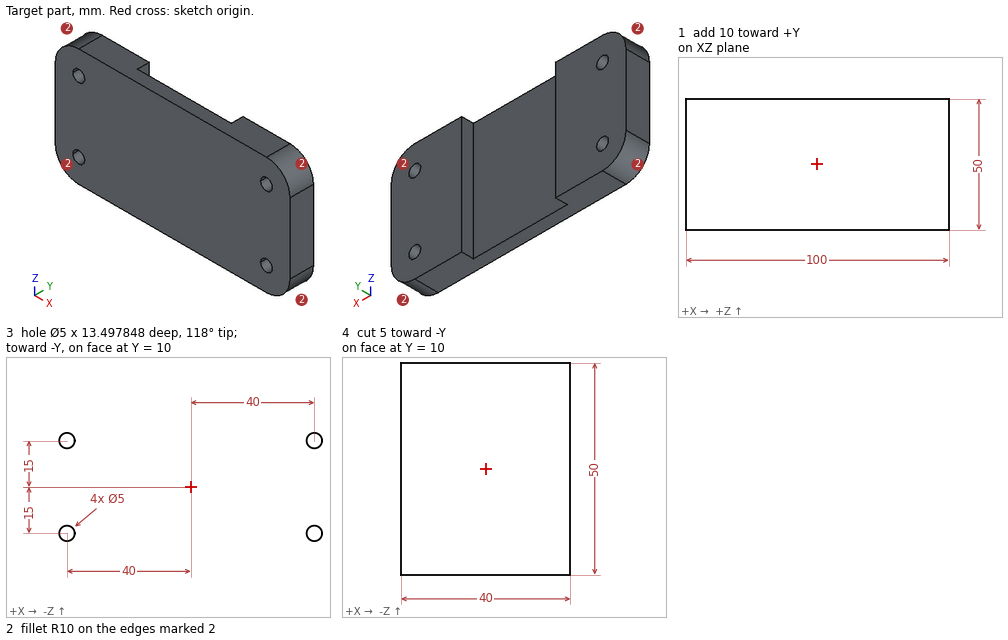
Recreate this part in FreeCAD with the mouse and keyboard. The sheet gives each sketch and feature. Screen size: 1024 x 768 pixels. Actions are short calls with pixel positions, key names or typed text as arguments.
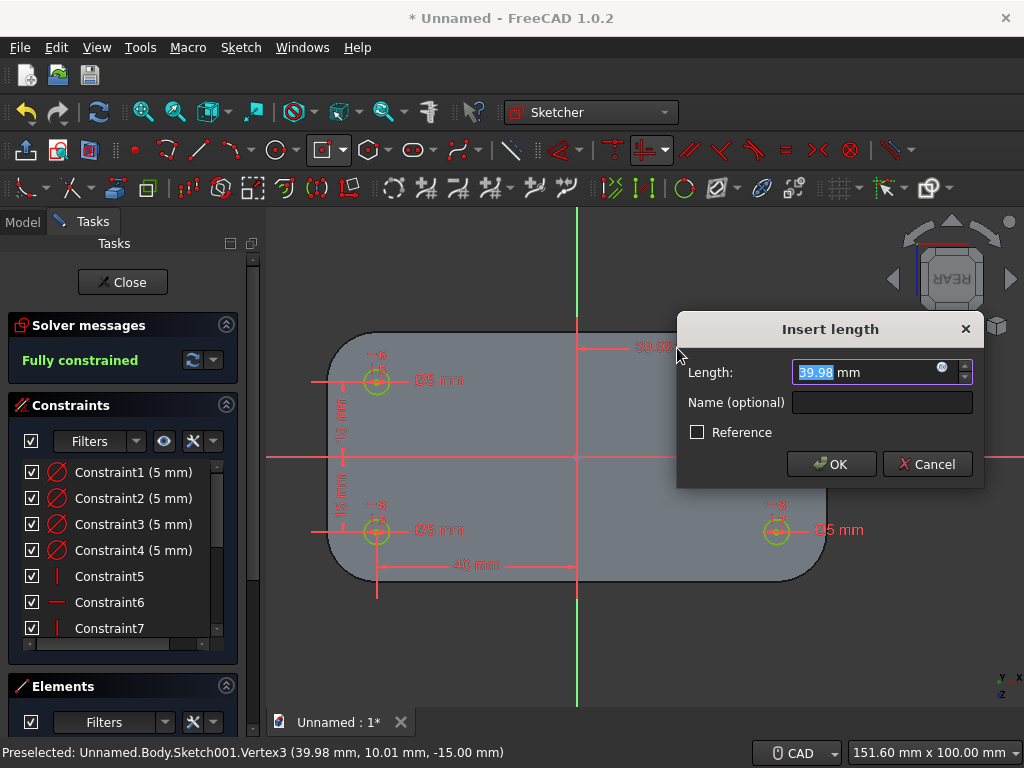
text(40)
key(Return)
key(Escape)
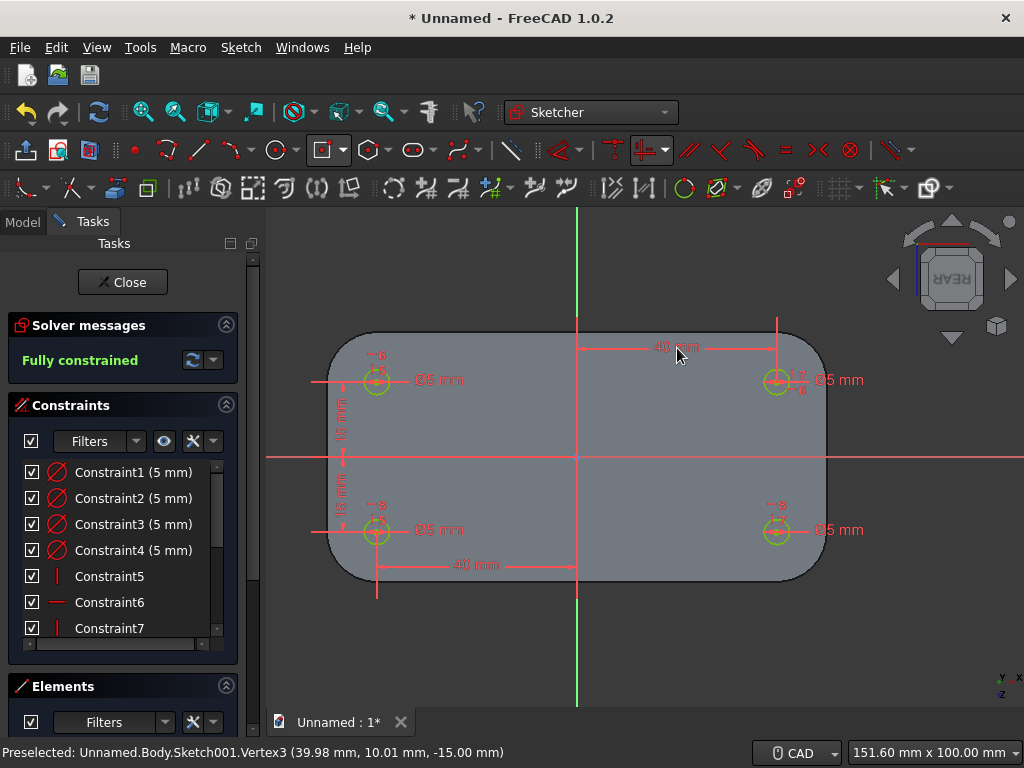
click(123, 282)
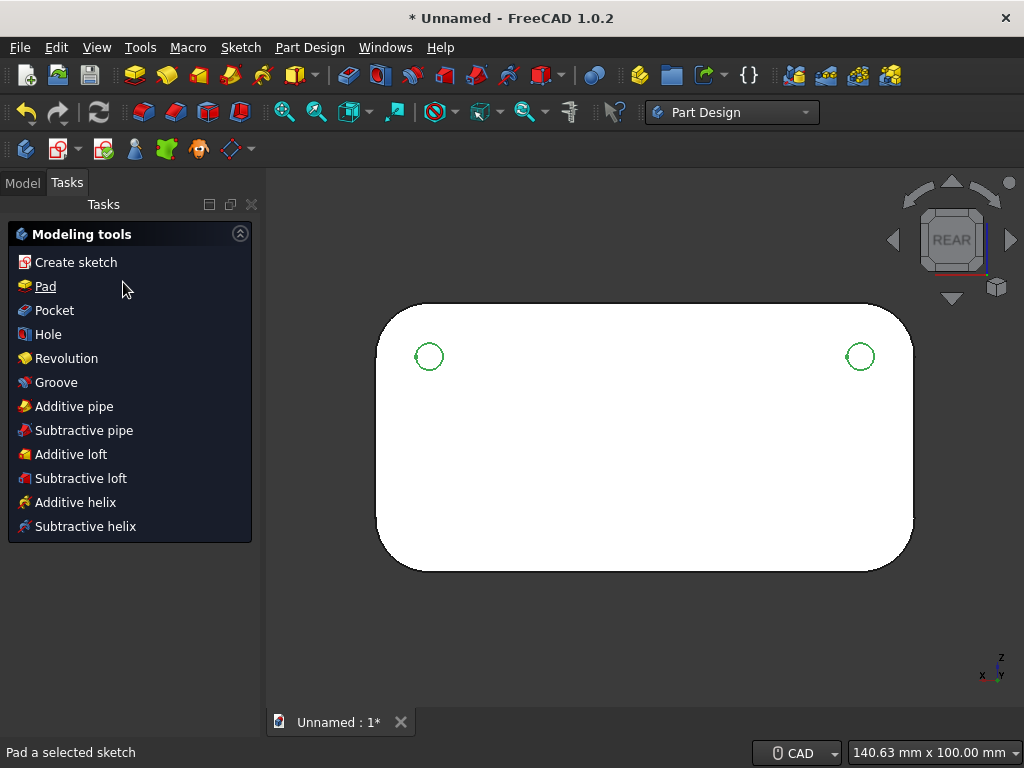
click(382, 76)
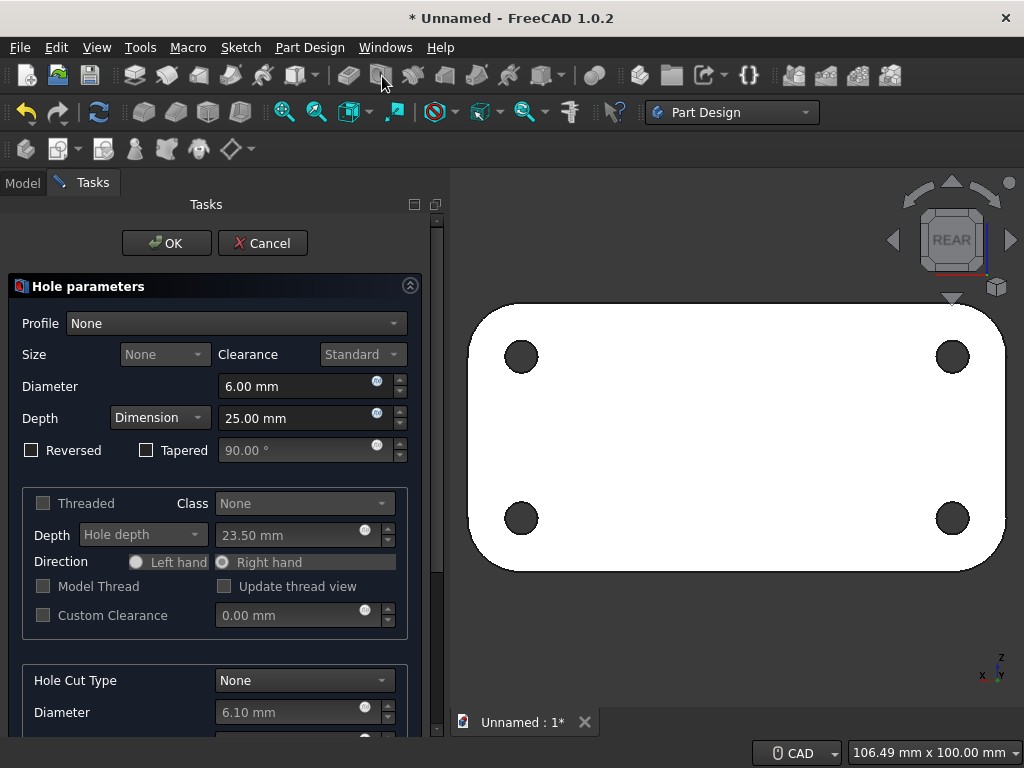
triple_click(305, 386)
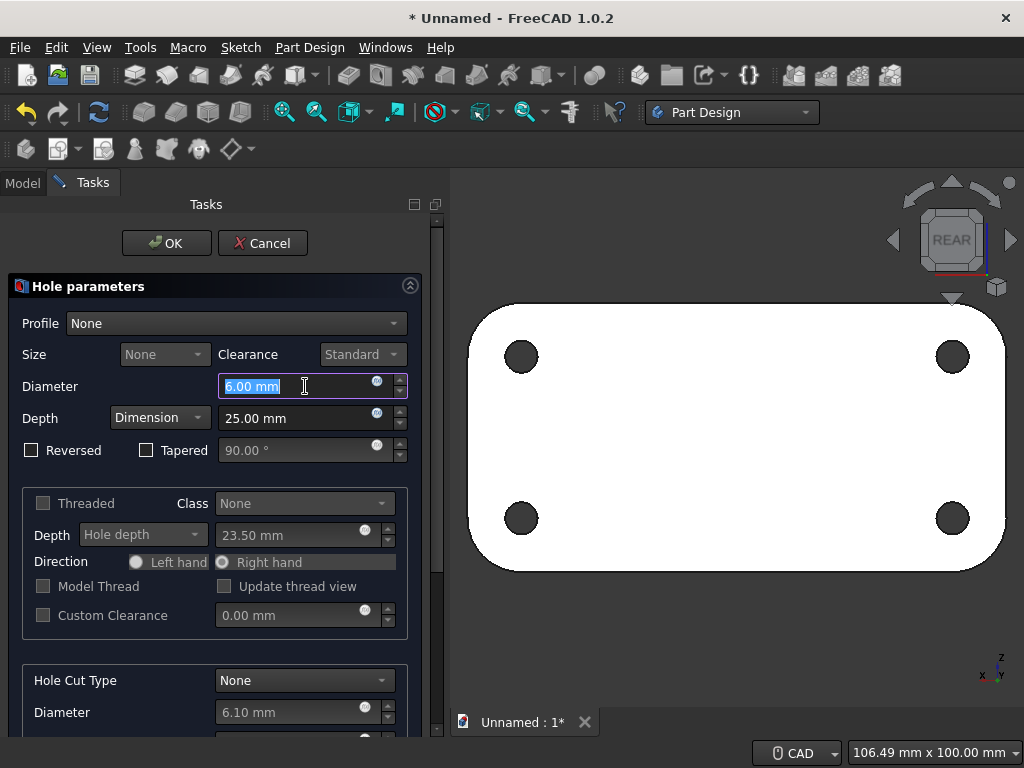
text(5)
key(Tab)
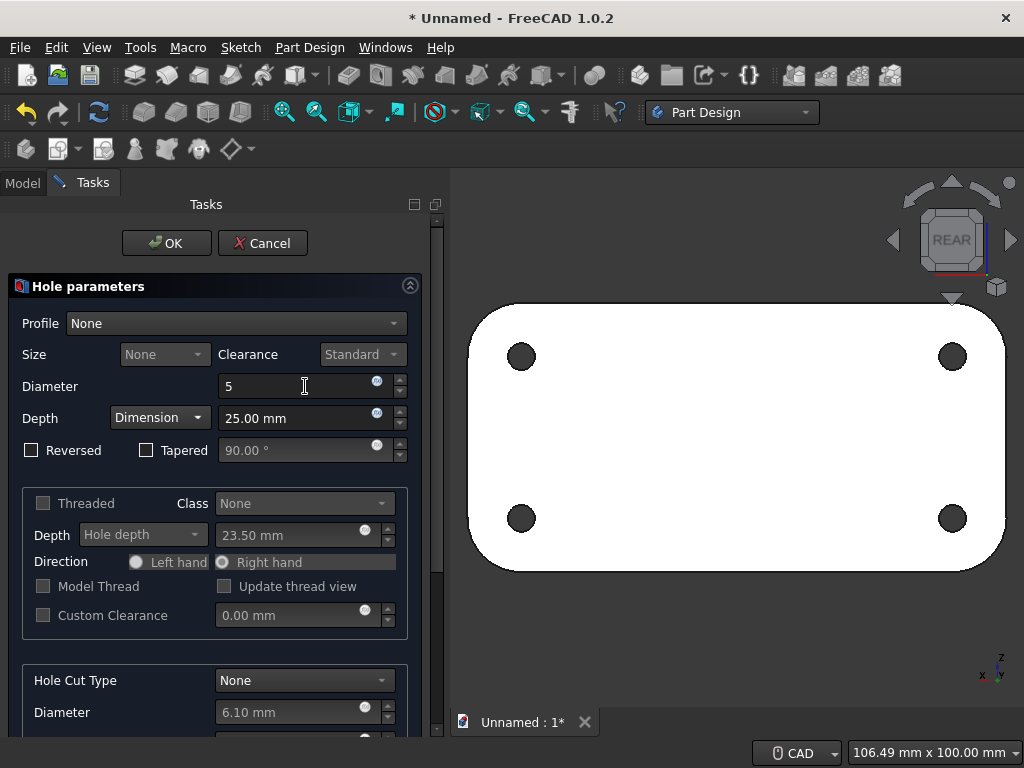
triple_click(305, 418)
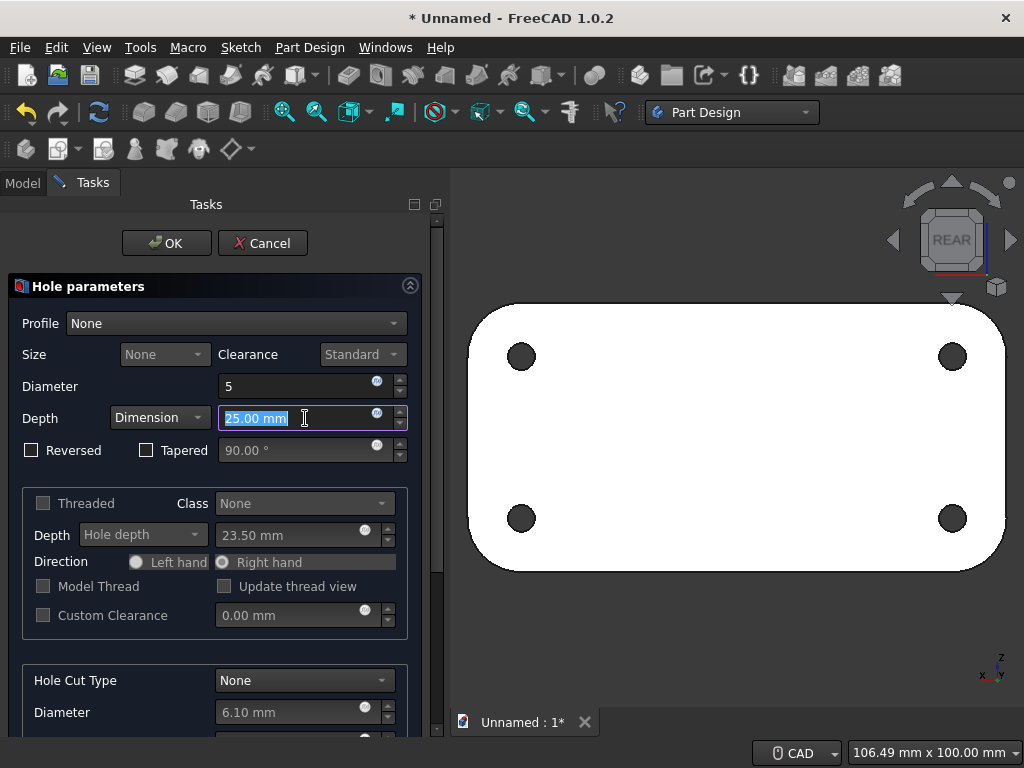
text(13.497848)
key(Tab)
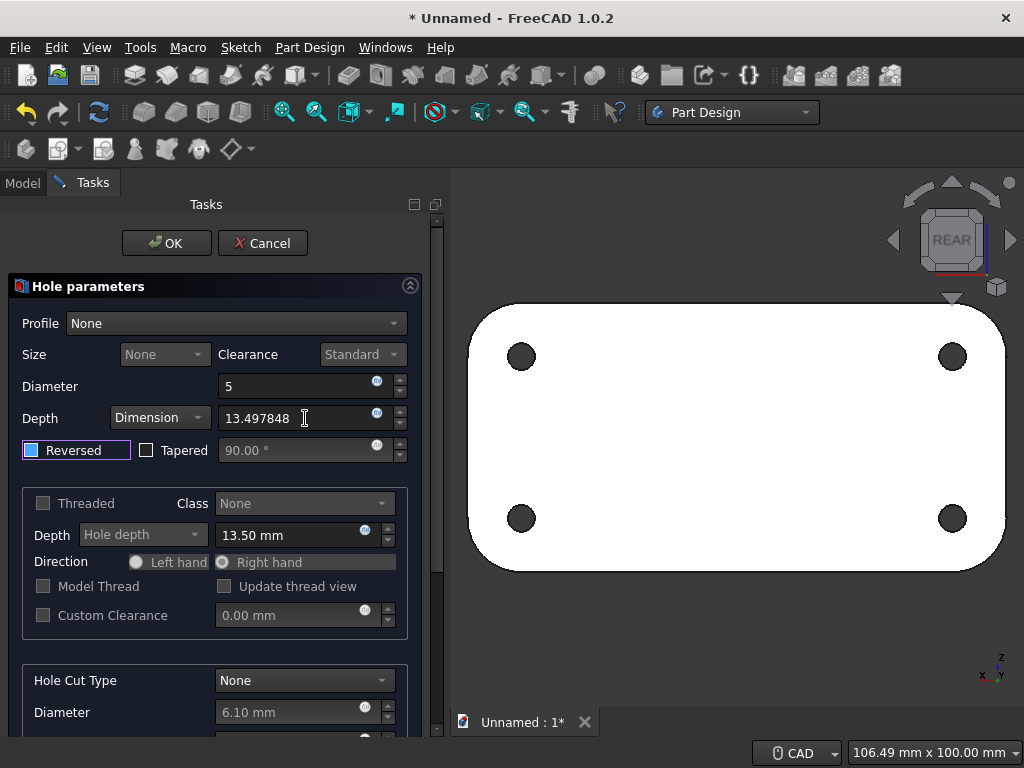
click(167, 243)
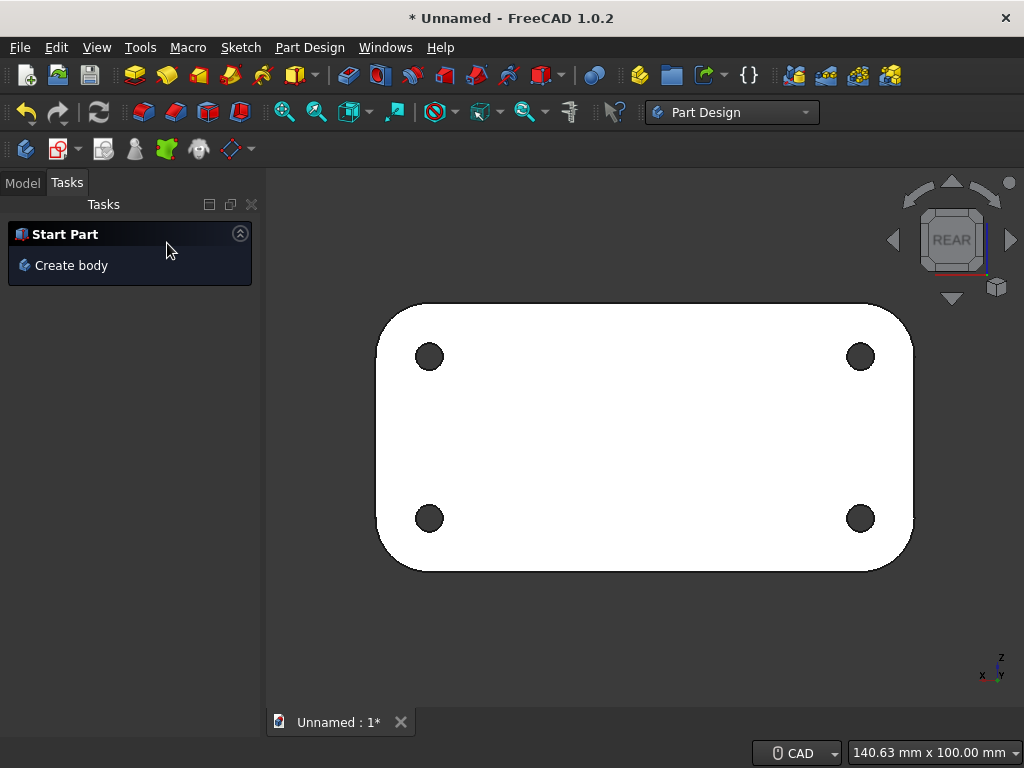
click(568, 436)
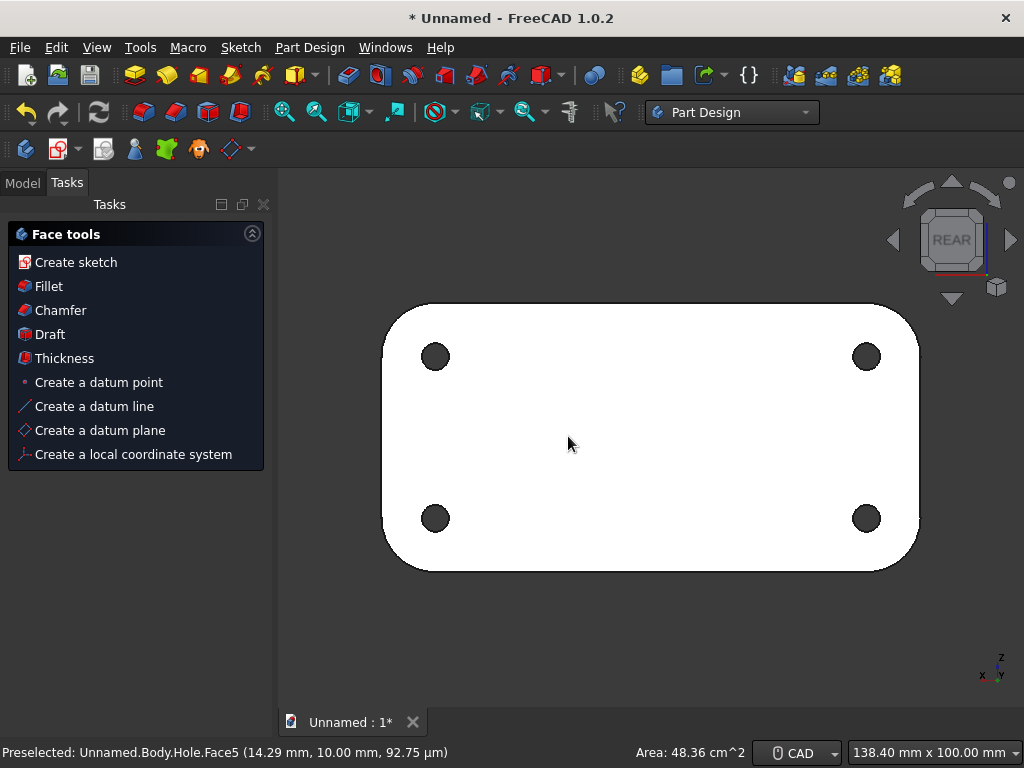
click(58, 150)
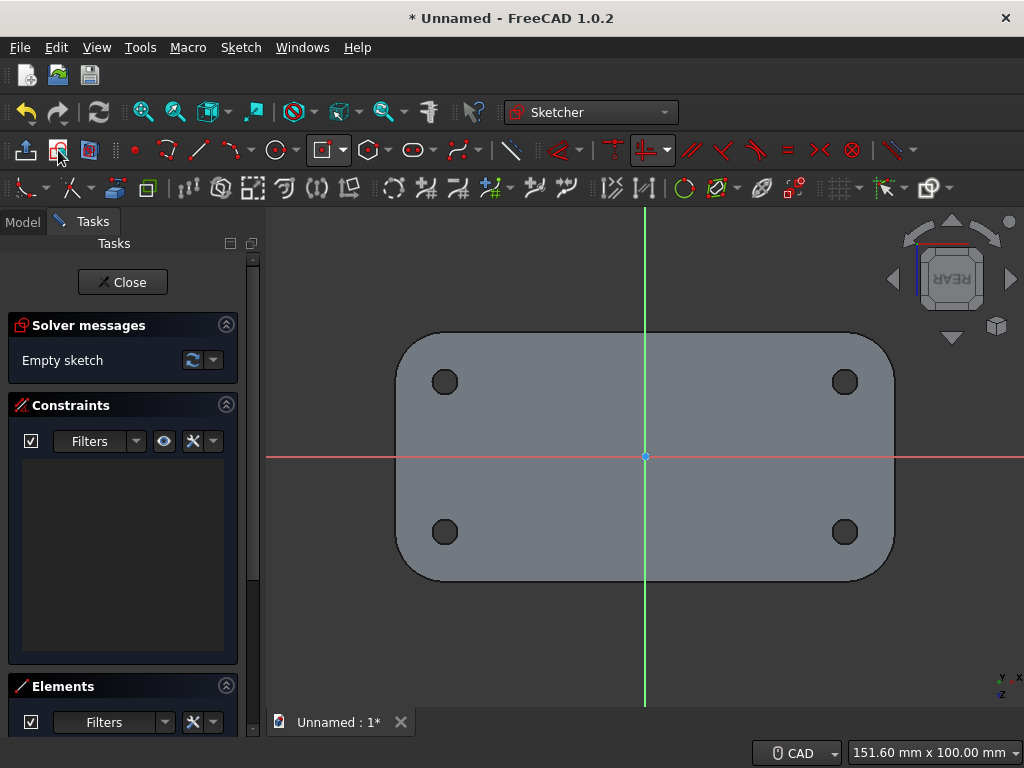
click(322, 150)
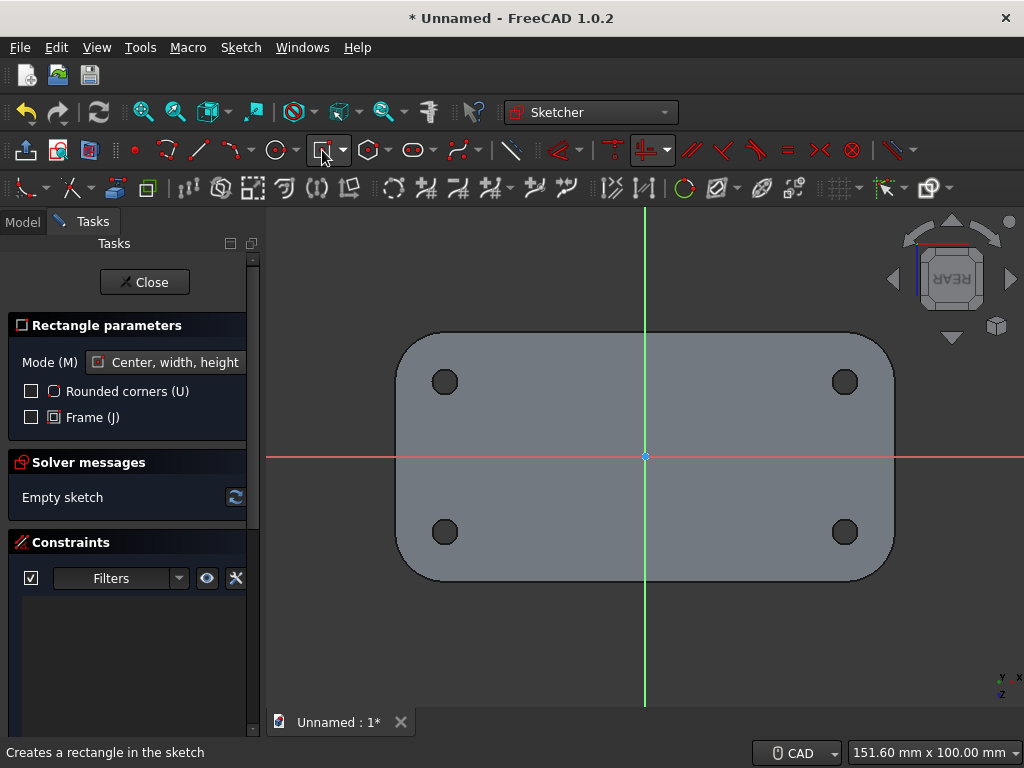
click(645, 457)
move(745, 332)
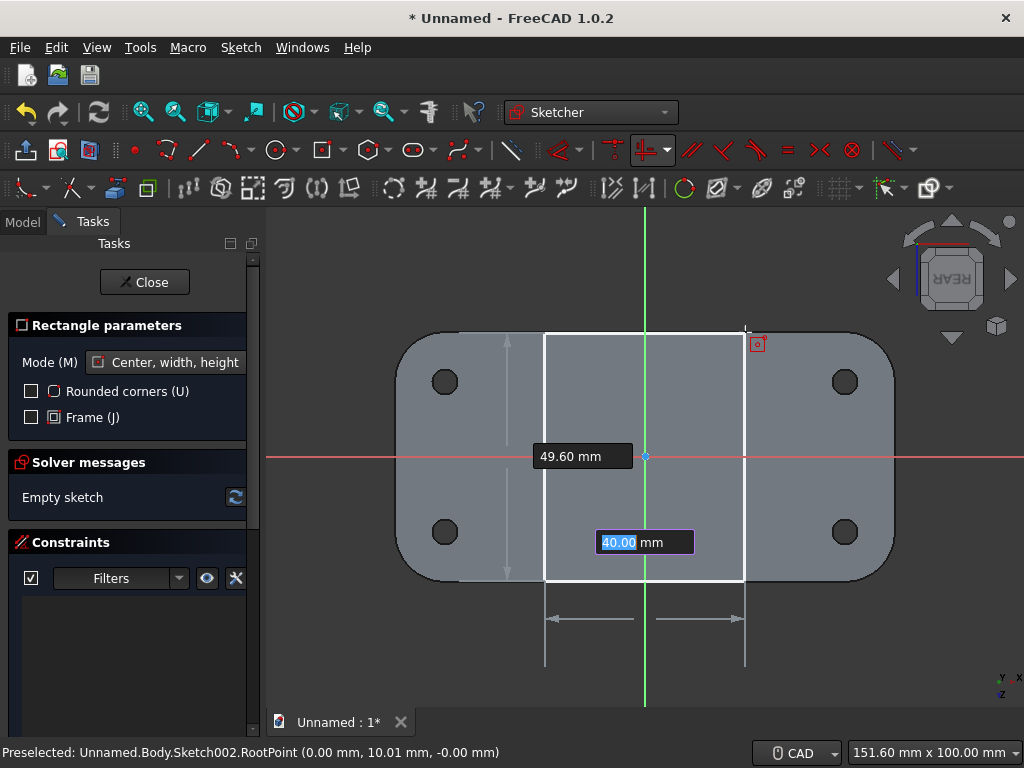
text(40)
key(Tab)
text(50)
key(Return)
key(Escape)